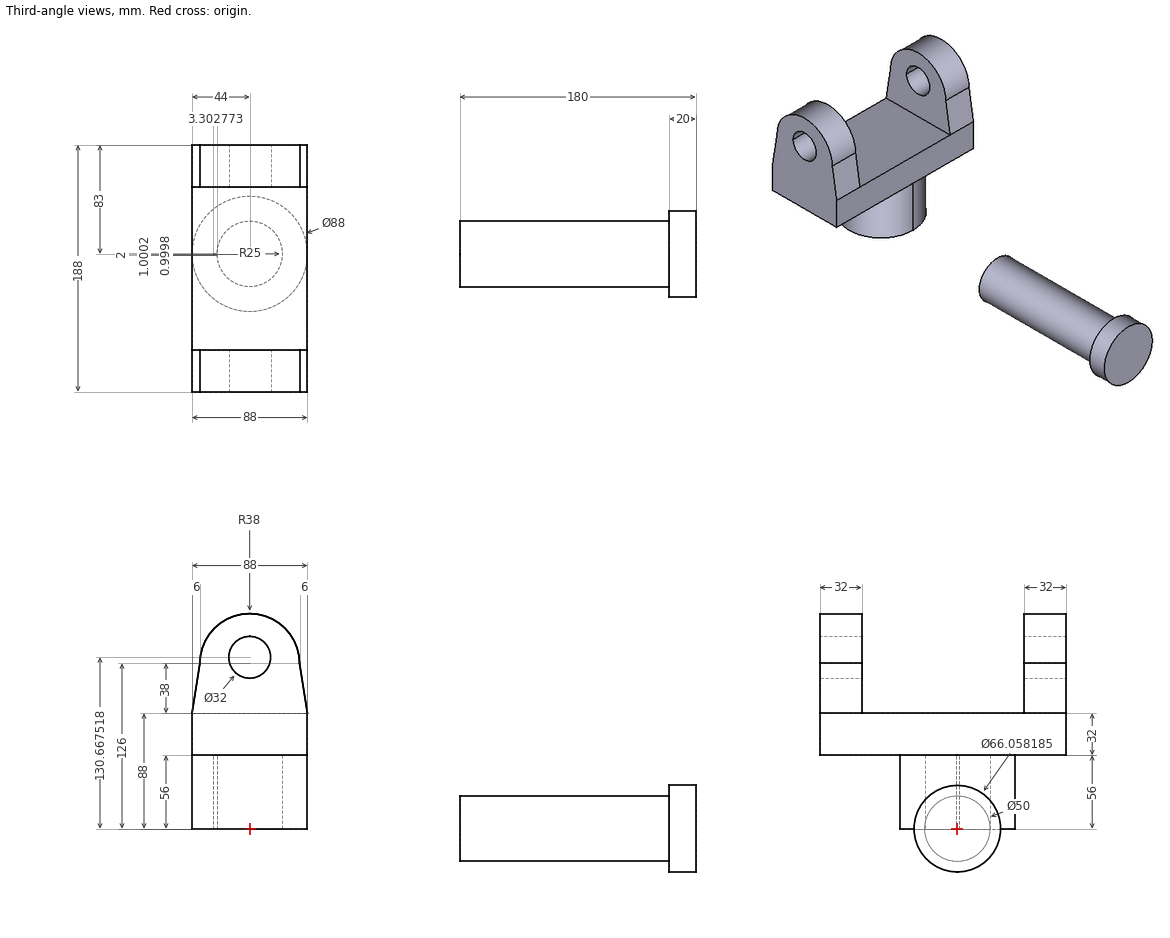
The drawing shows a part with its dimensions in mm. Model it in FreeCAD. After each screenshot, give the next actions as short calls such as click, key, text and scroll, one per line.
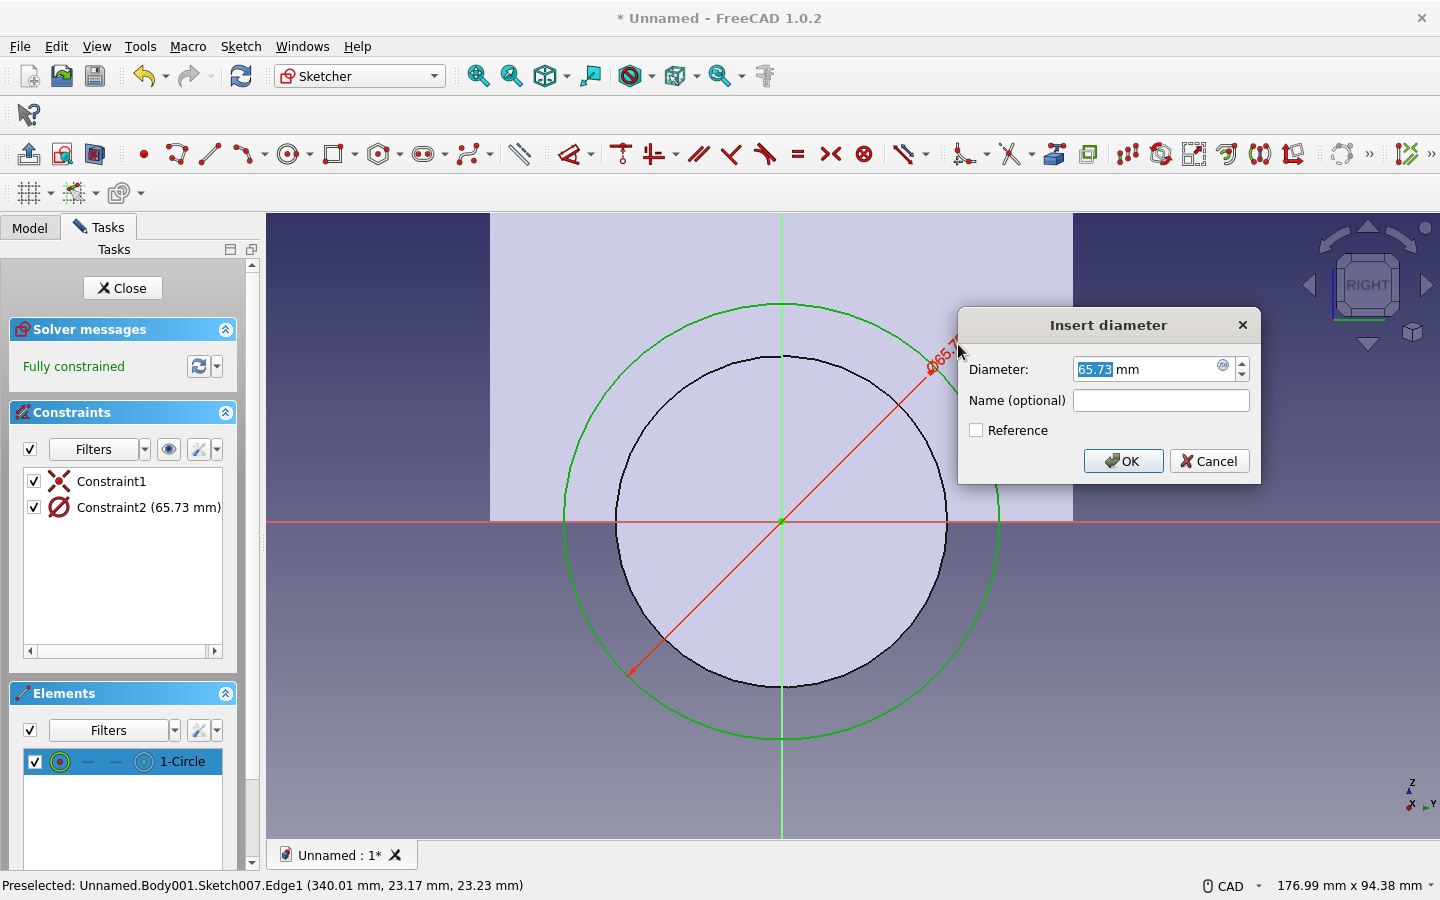
text(66.058185)
key(Return)
key(Escape)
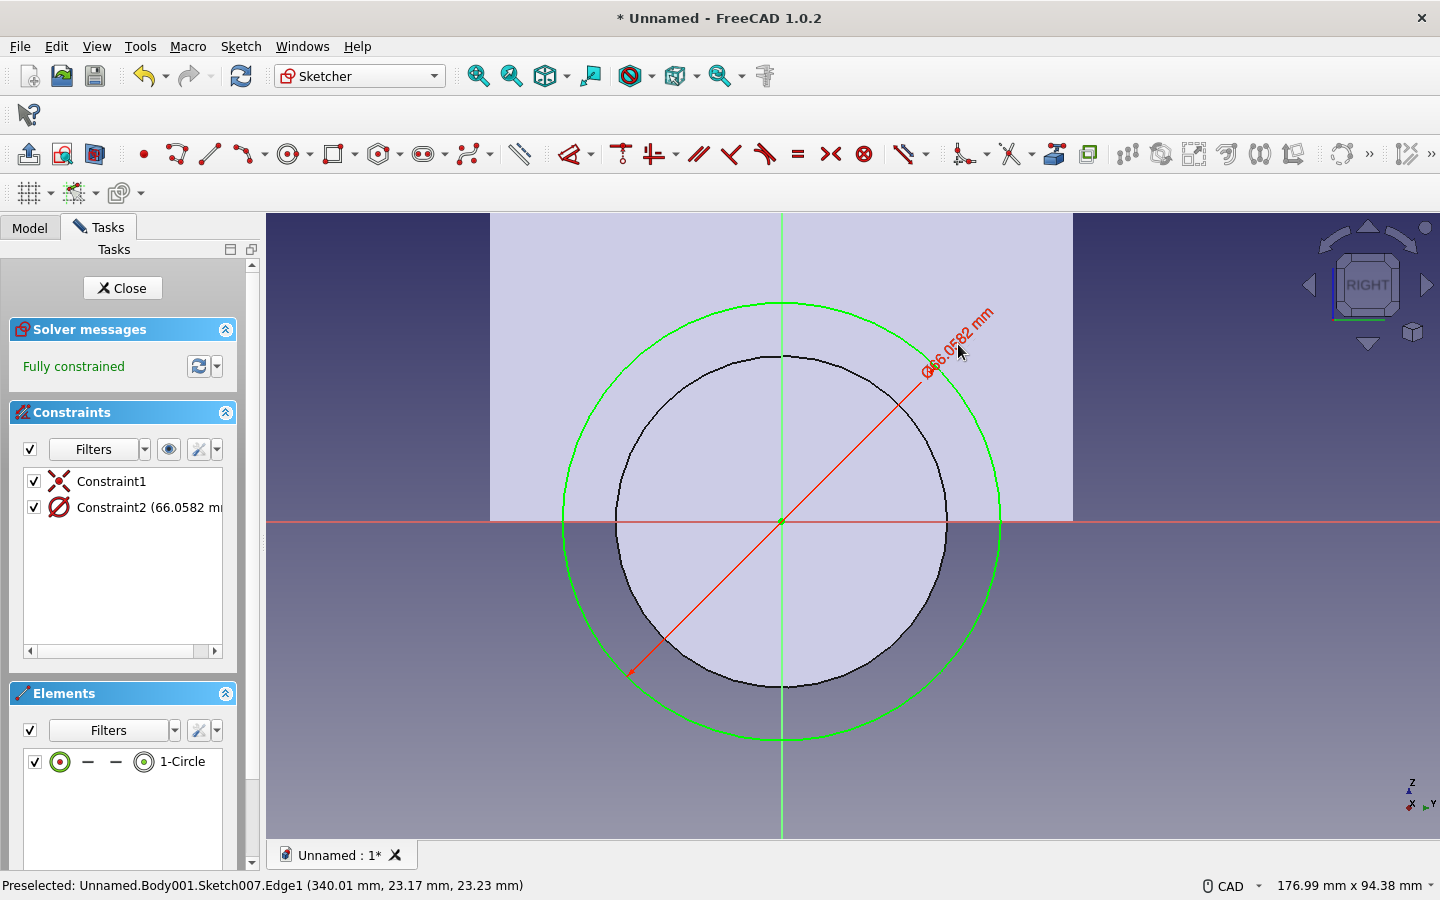
click(123, 288)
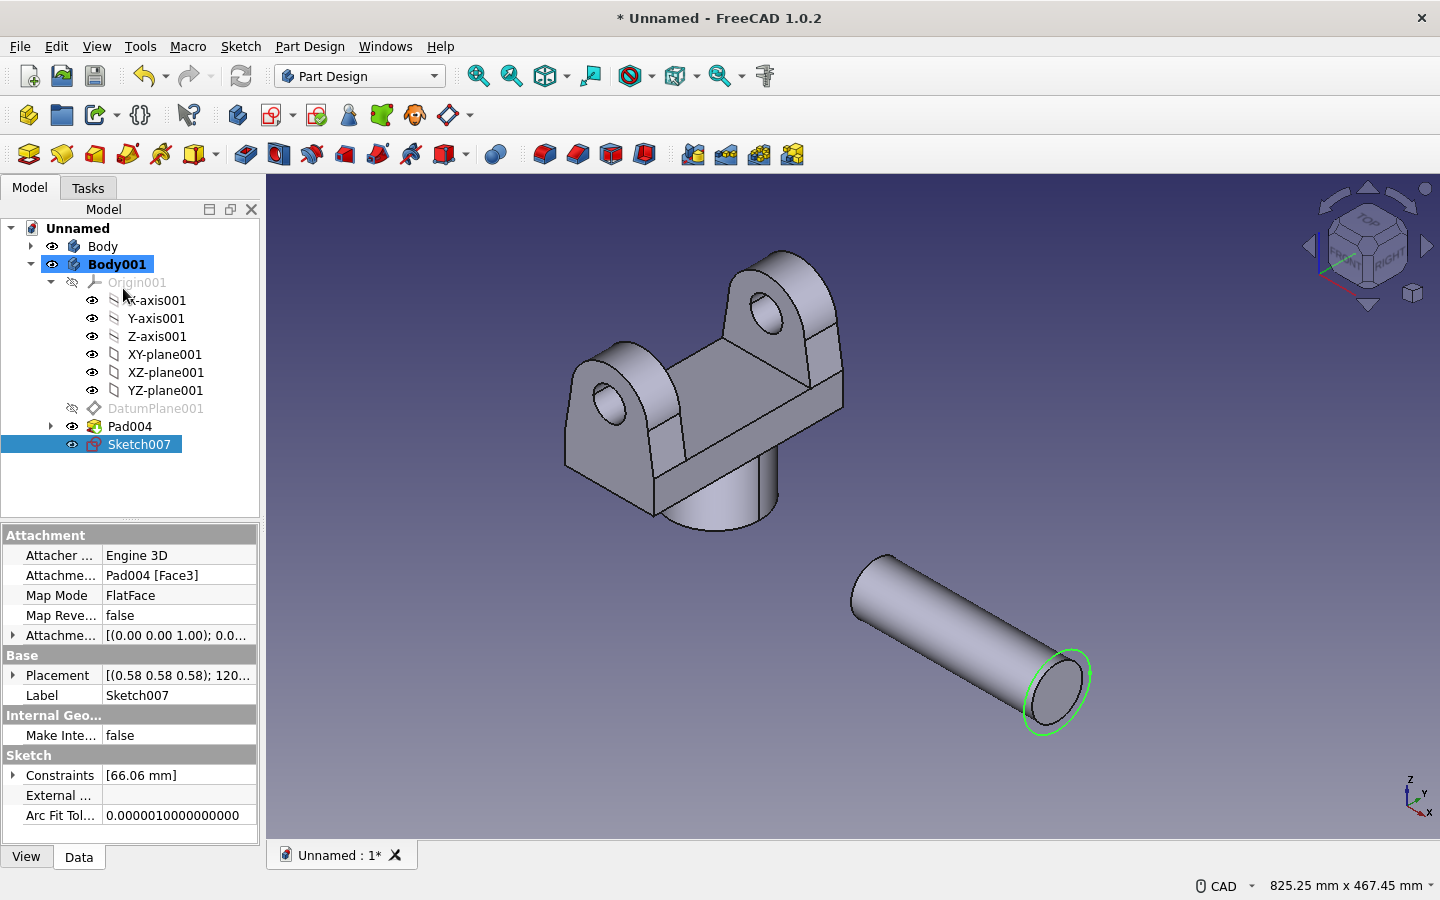
click(29, 154)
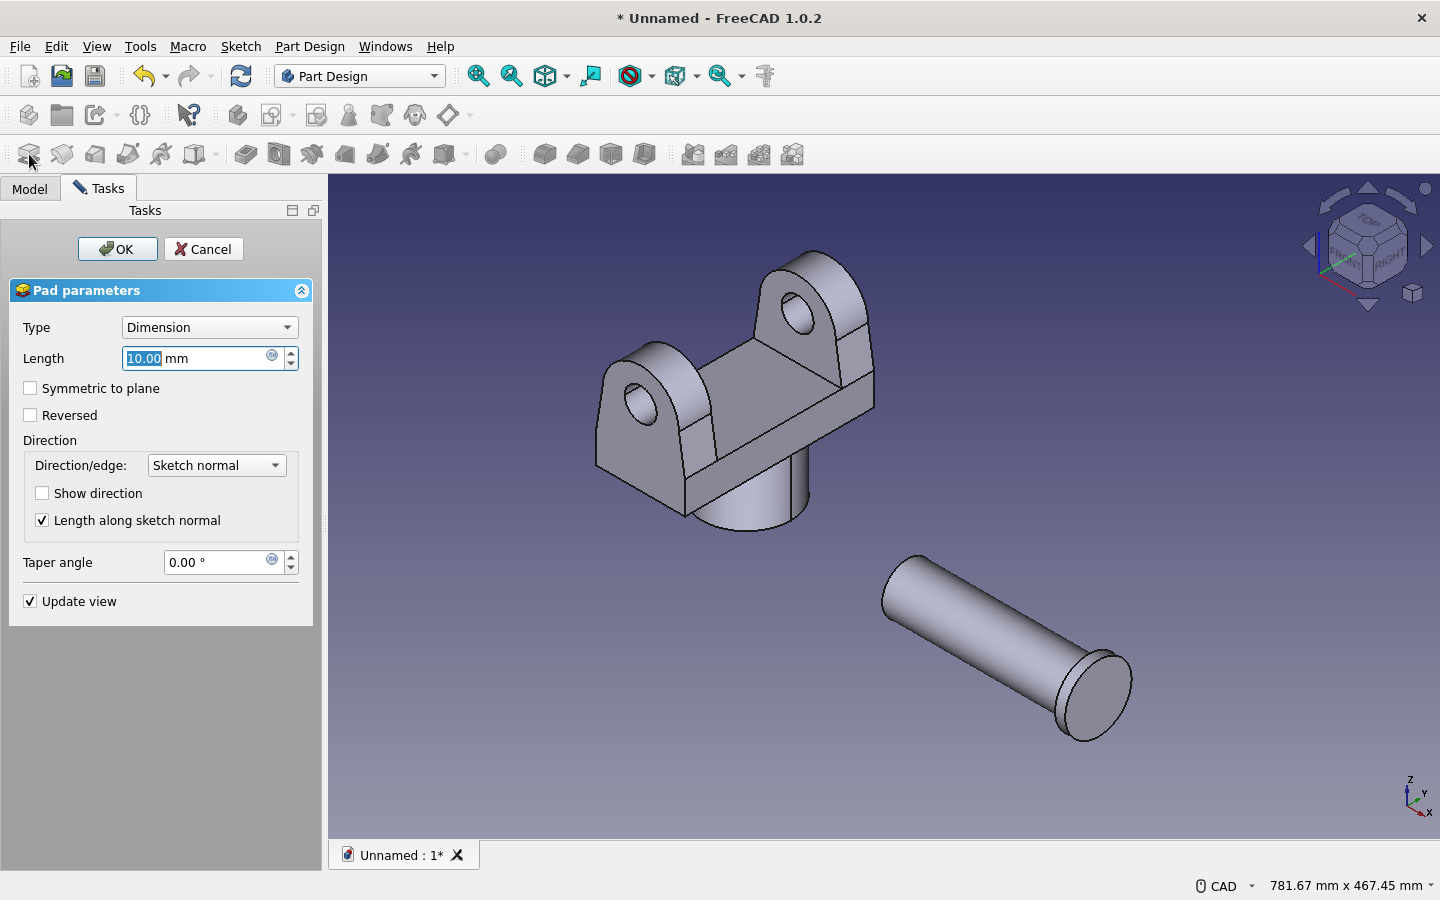
text(20)
key(Tab)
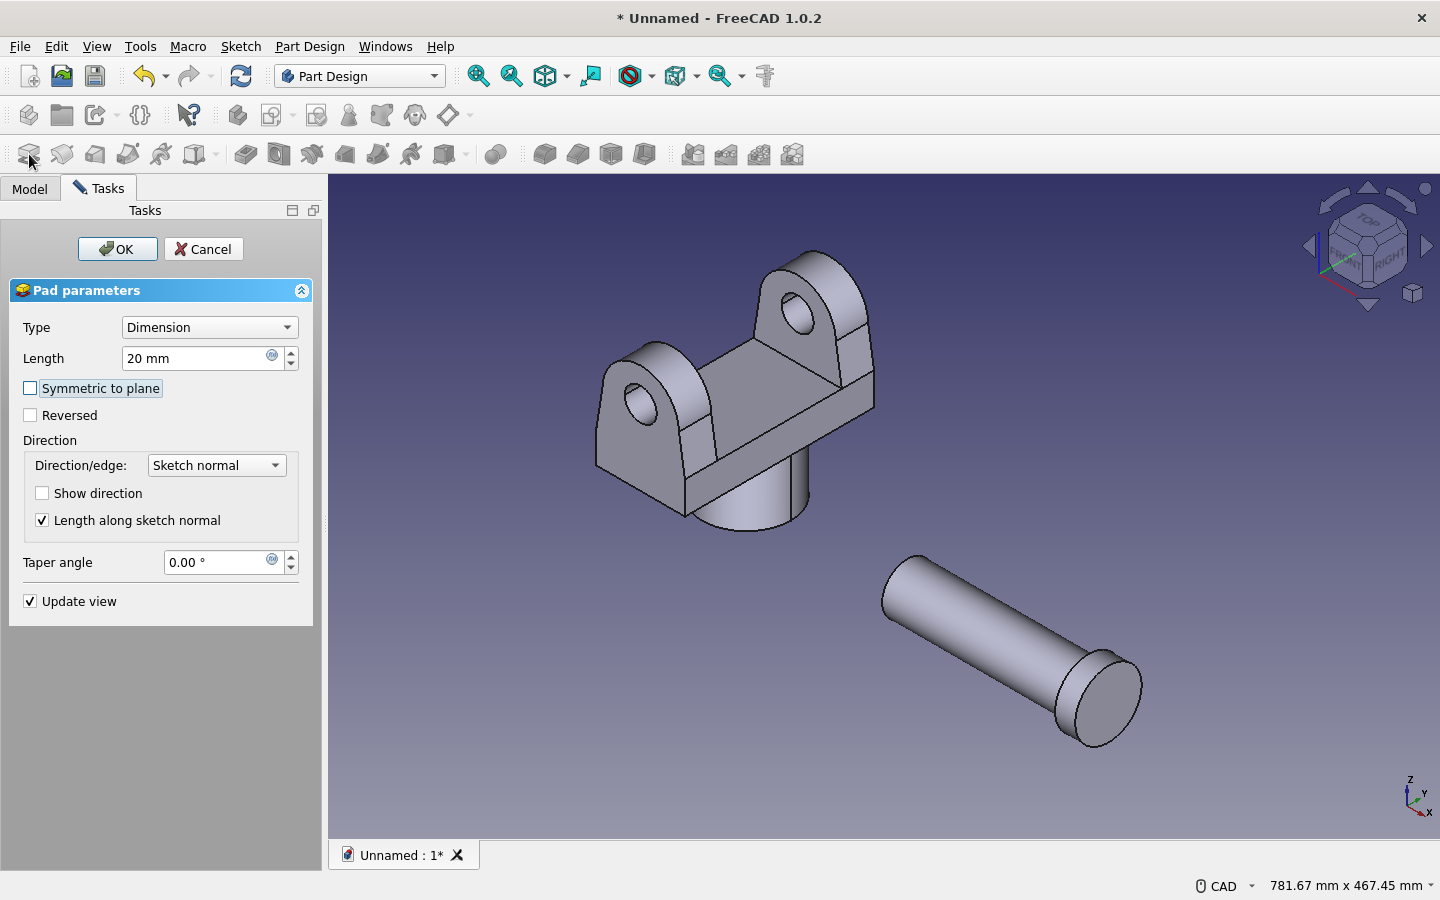
click(31, 415)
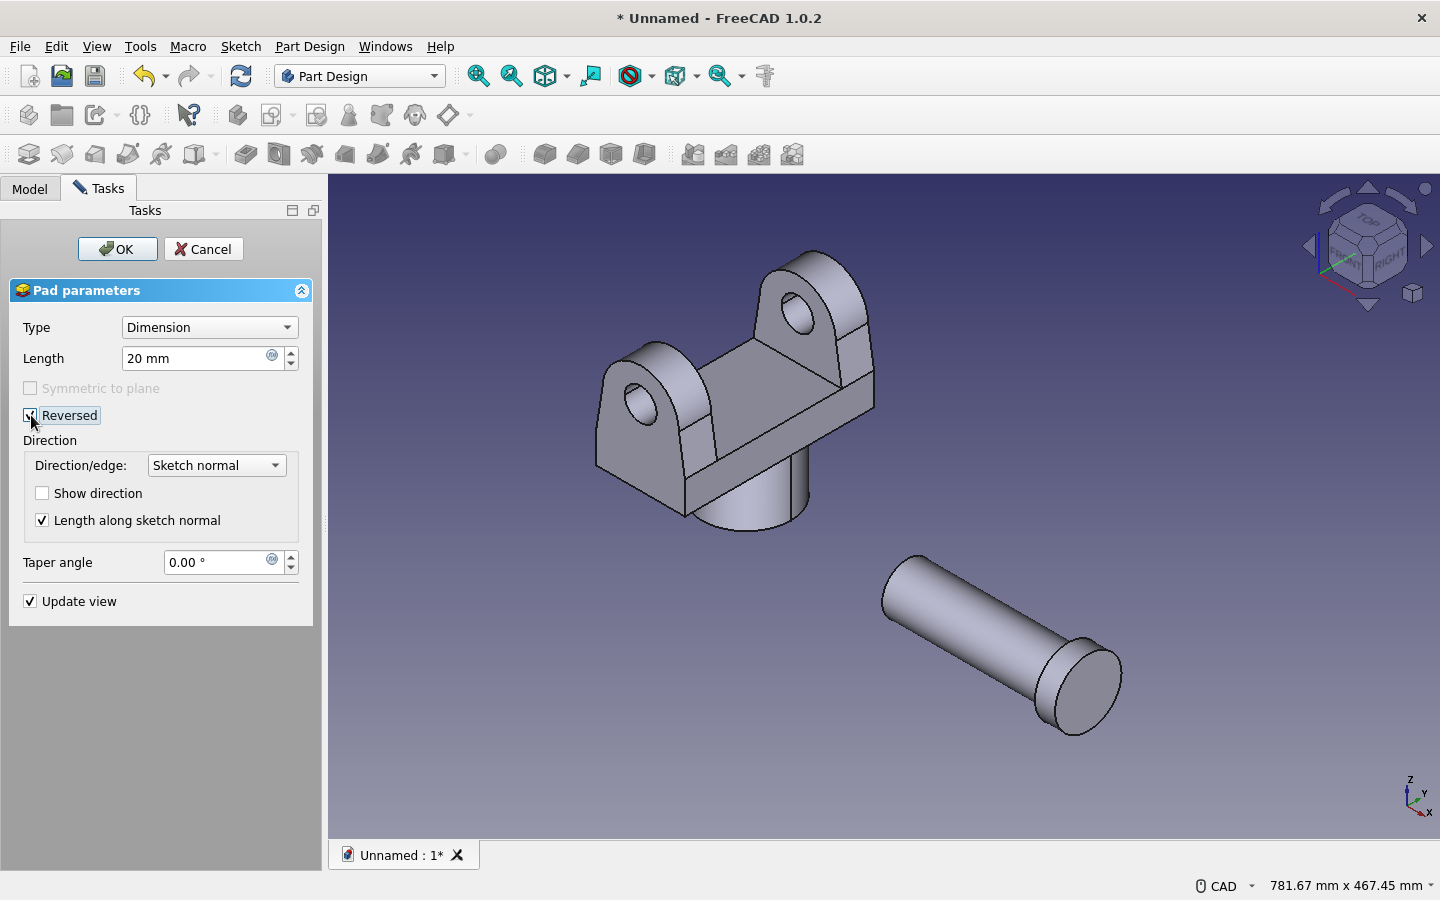
click(118, 249)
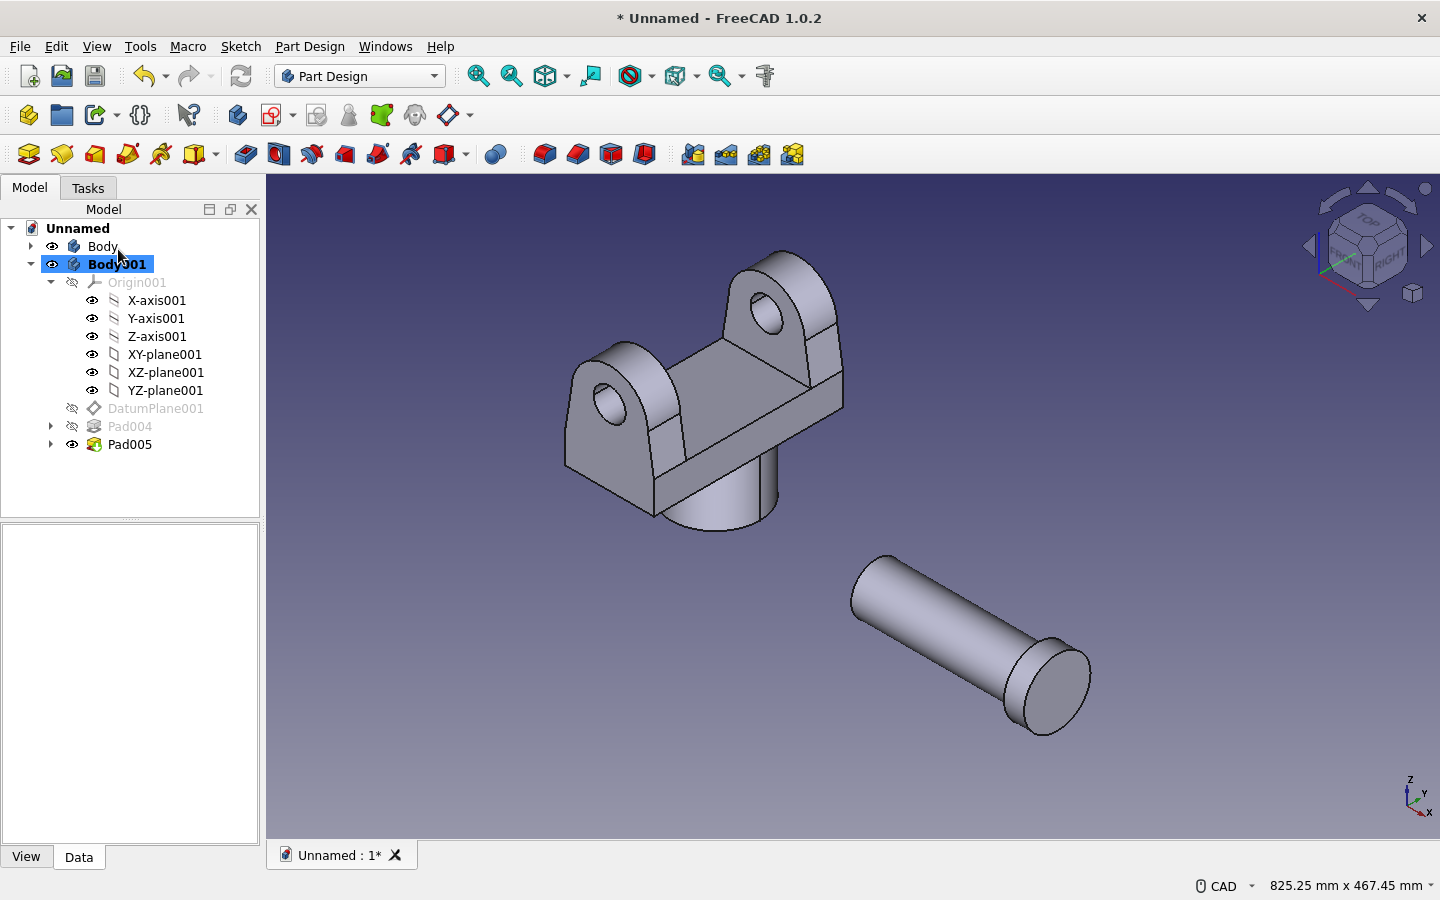
key(v)
key(f)